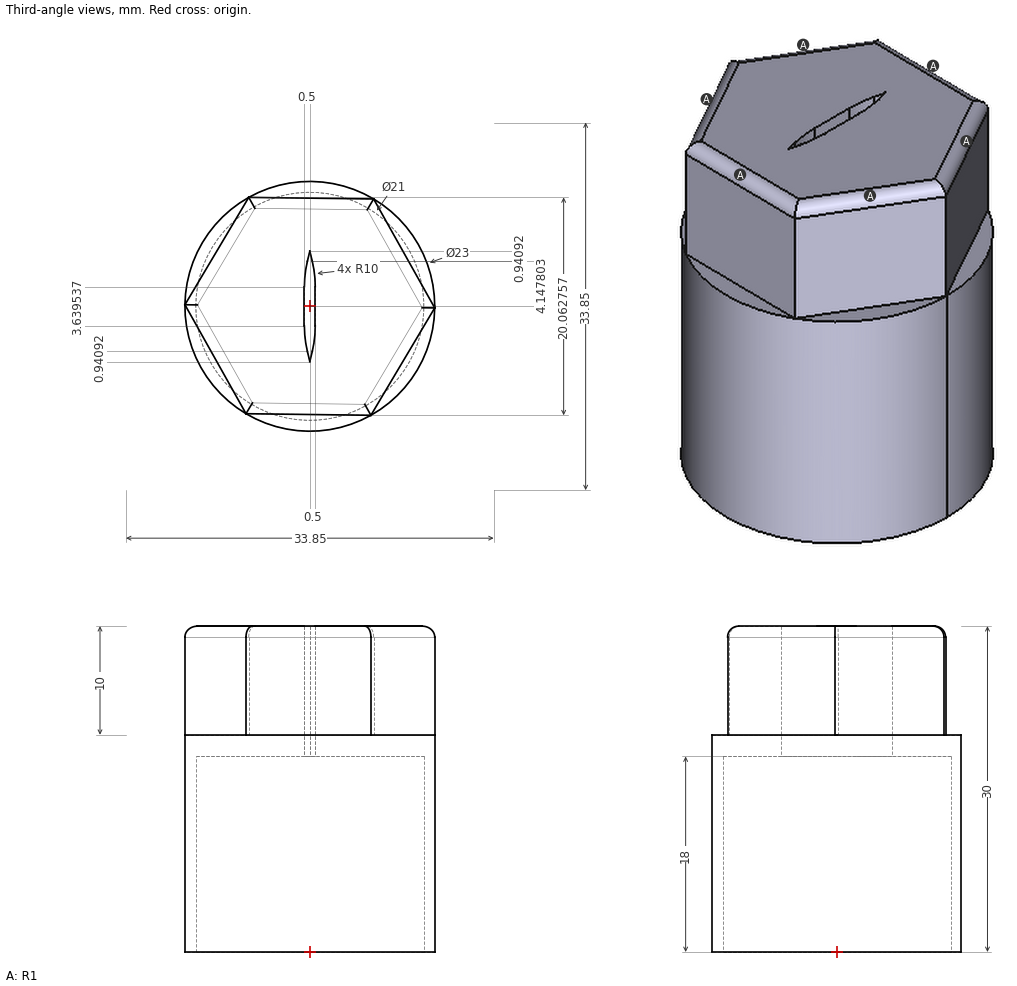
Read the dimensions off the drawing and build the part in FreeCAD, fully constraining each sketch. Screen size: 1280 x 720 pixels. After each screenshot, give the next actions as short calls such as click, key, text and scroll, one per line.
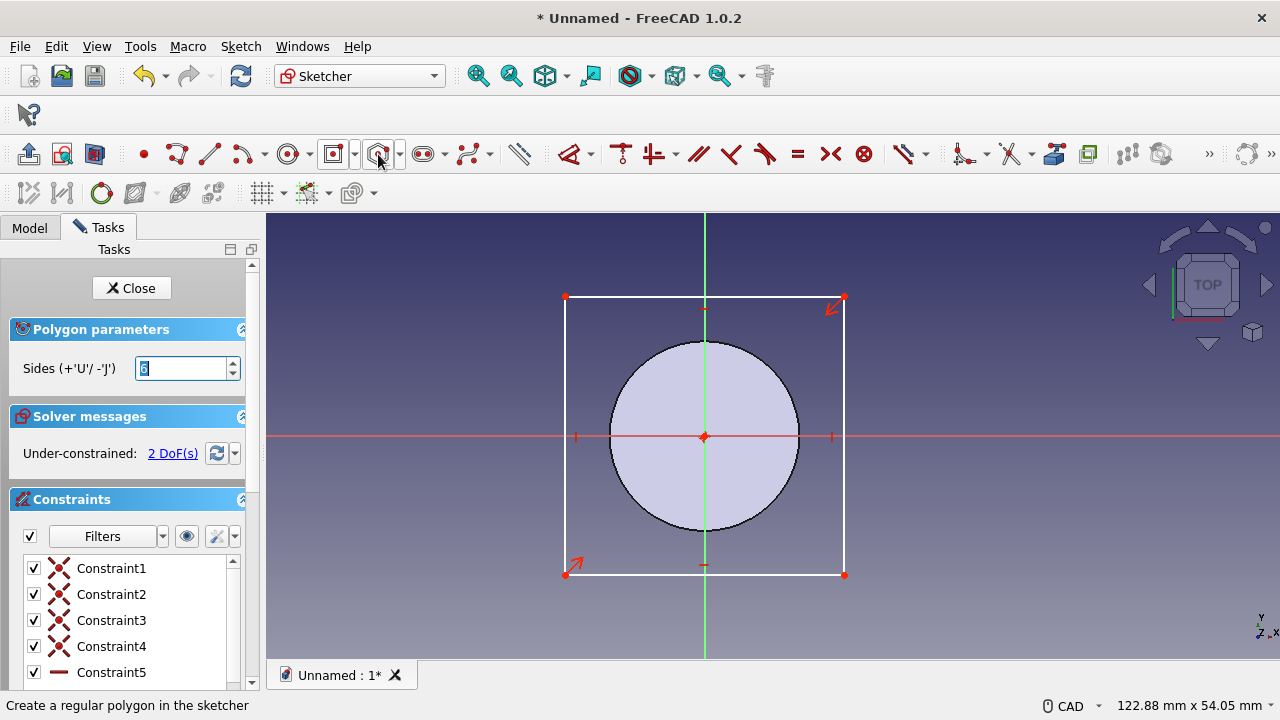
click(705, 436)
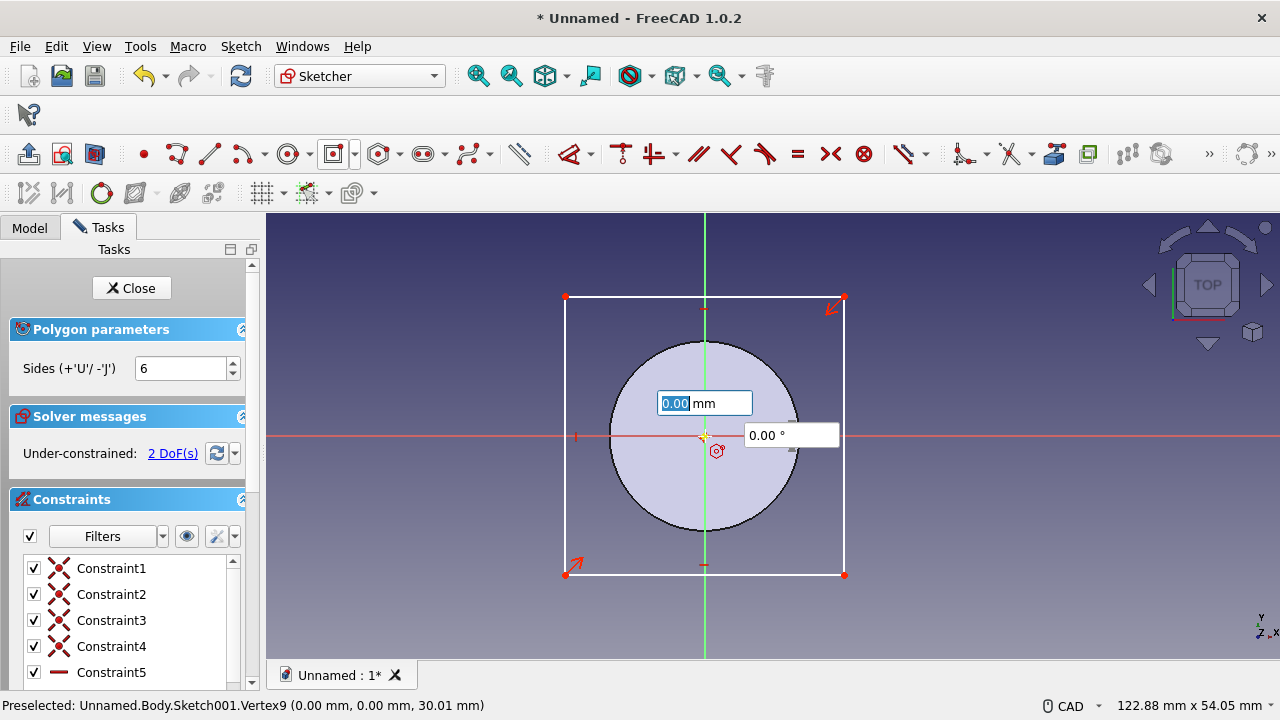
click(753, 355)
key(Escape)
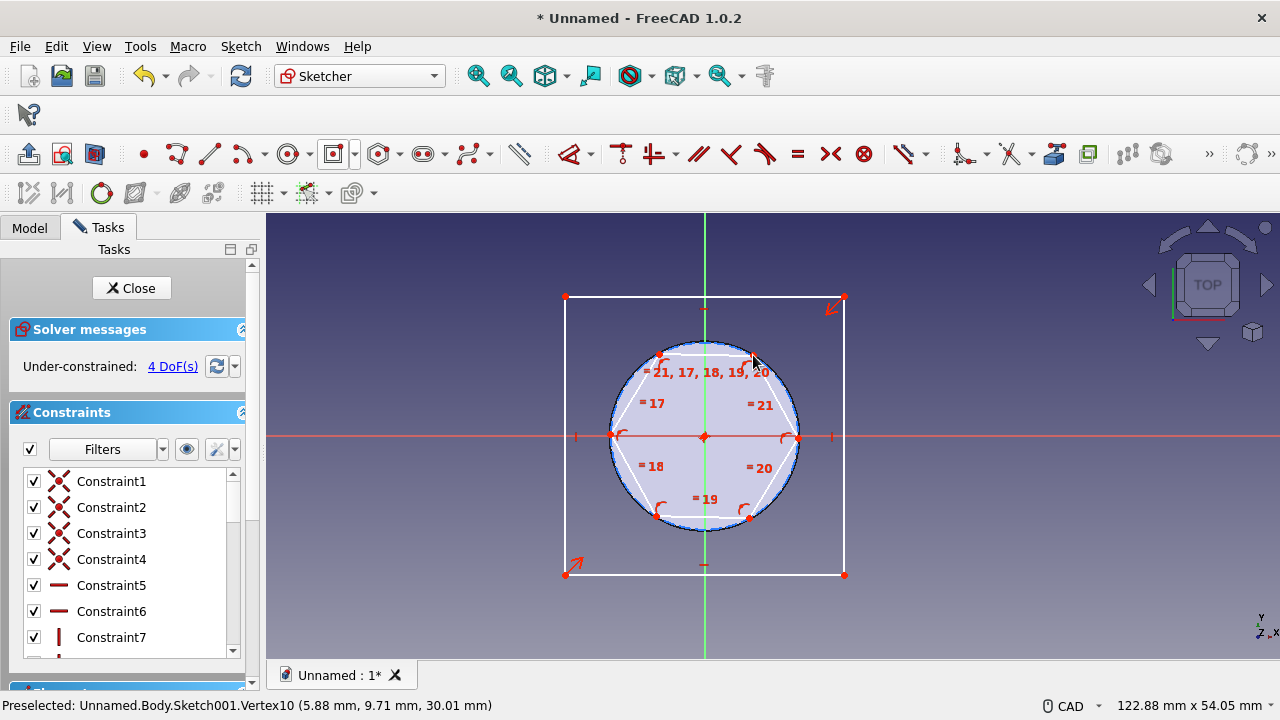
scroll(638, 370, up, 2)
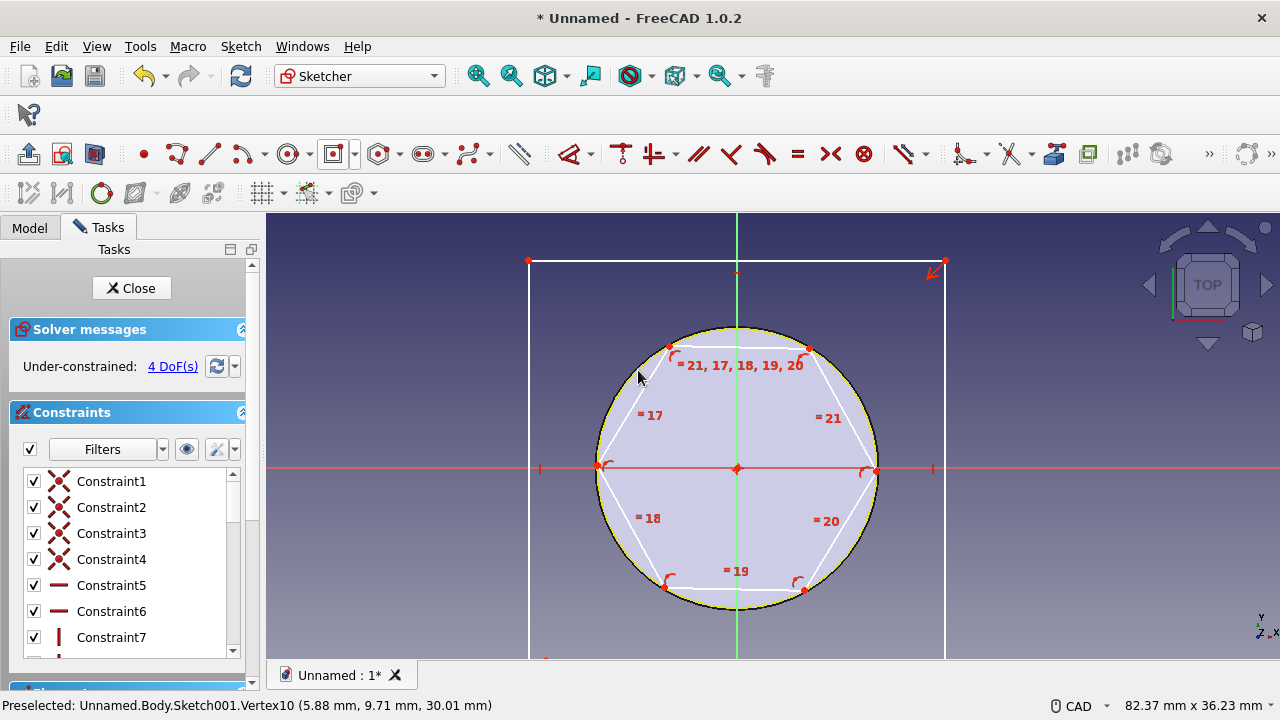
click(638, 370)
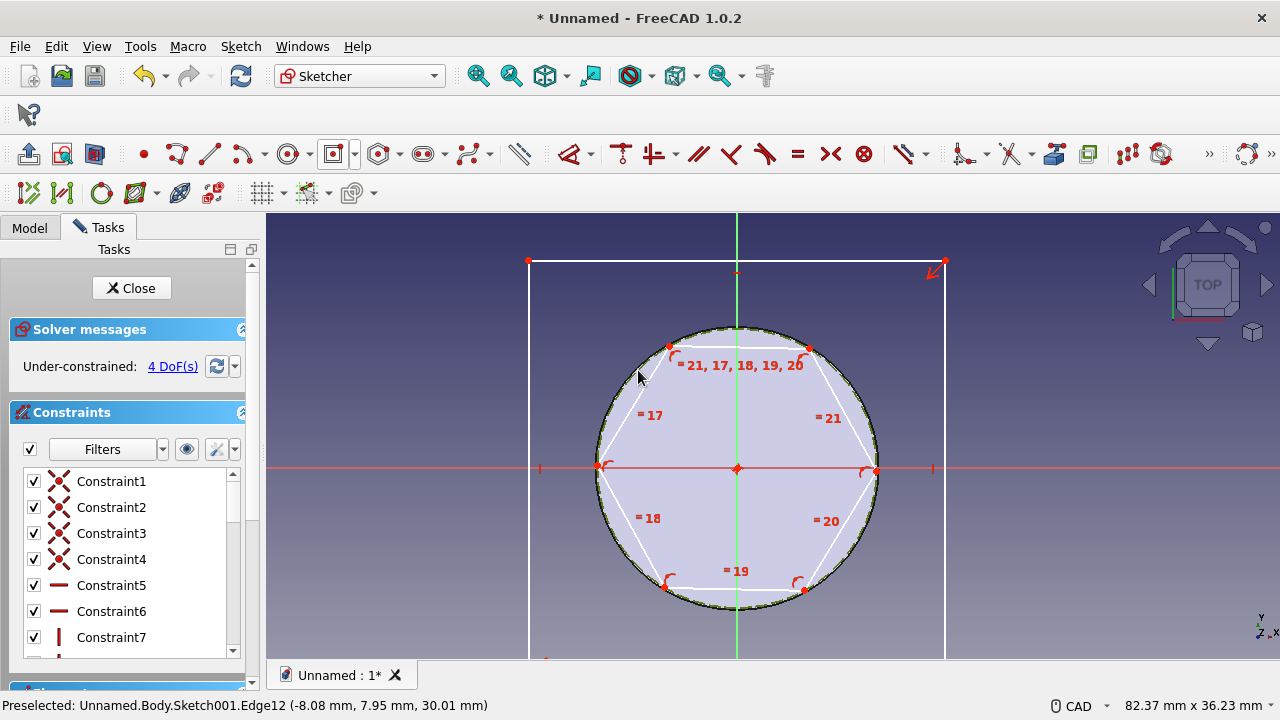
click(590, 154)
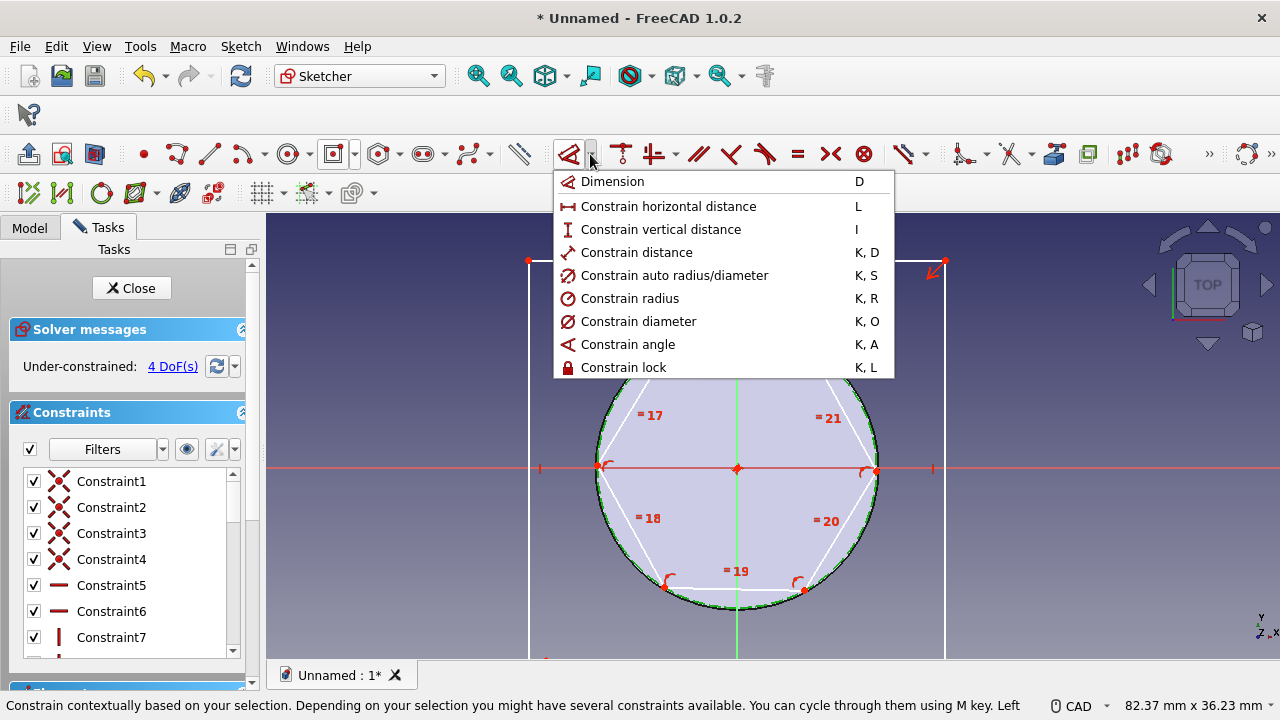
click(724, 322)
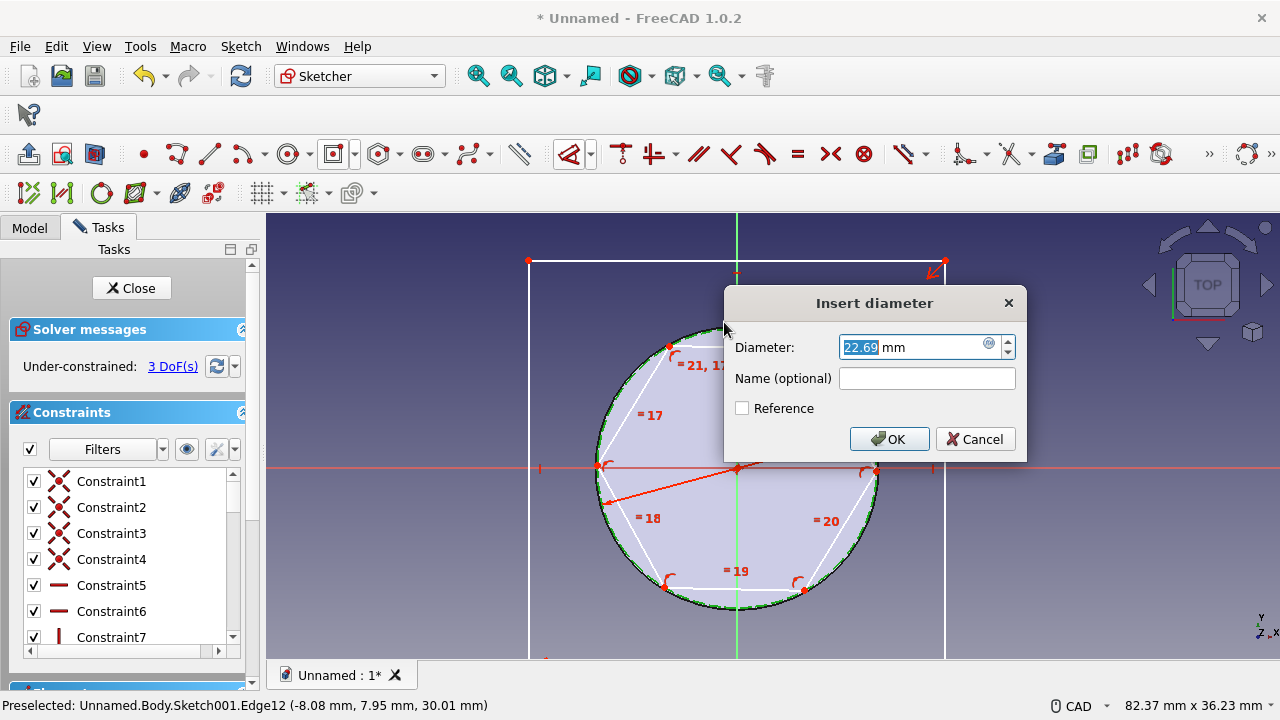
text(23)
key(Return)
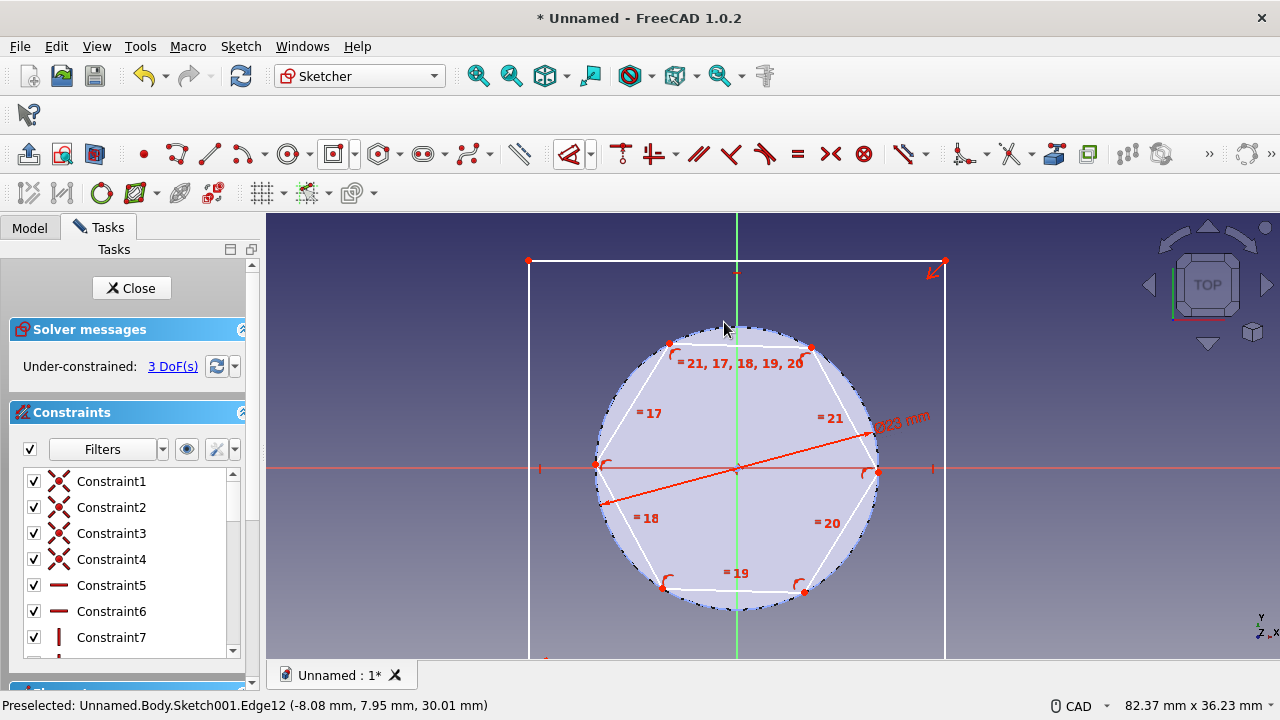
scroll(638, 370, down, 2)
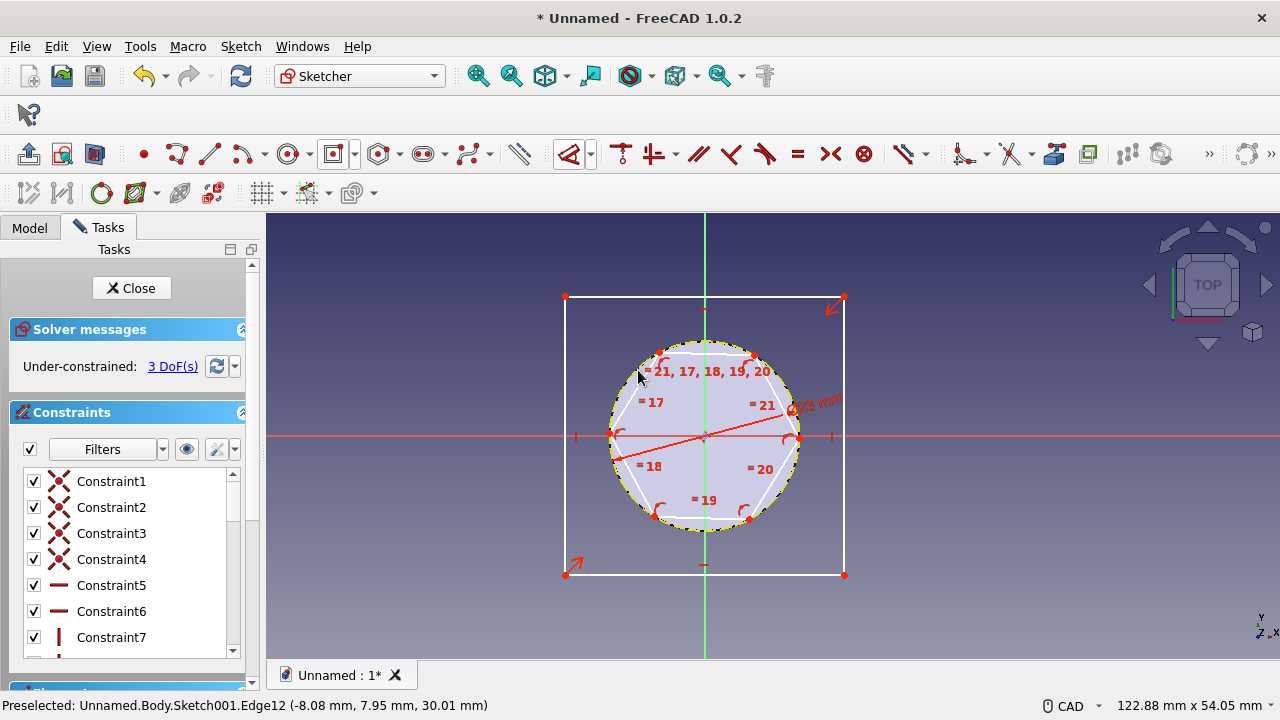
click(649, 575)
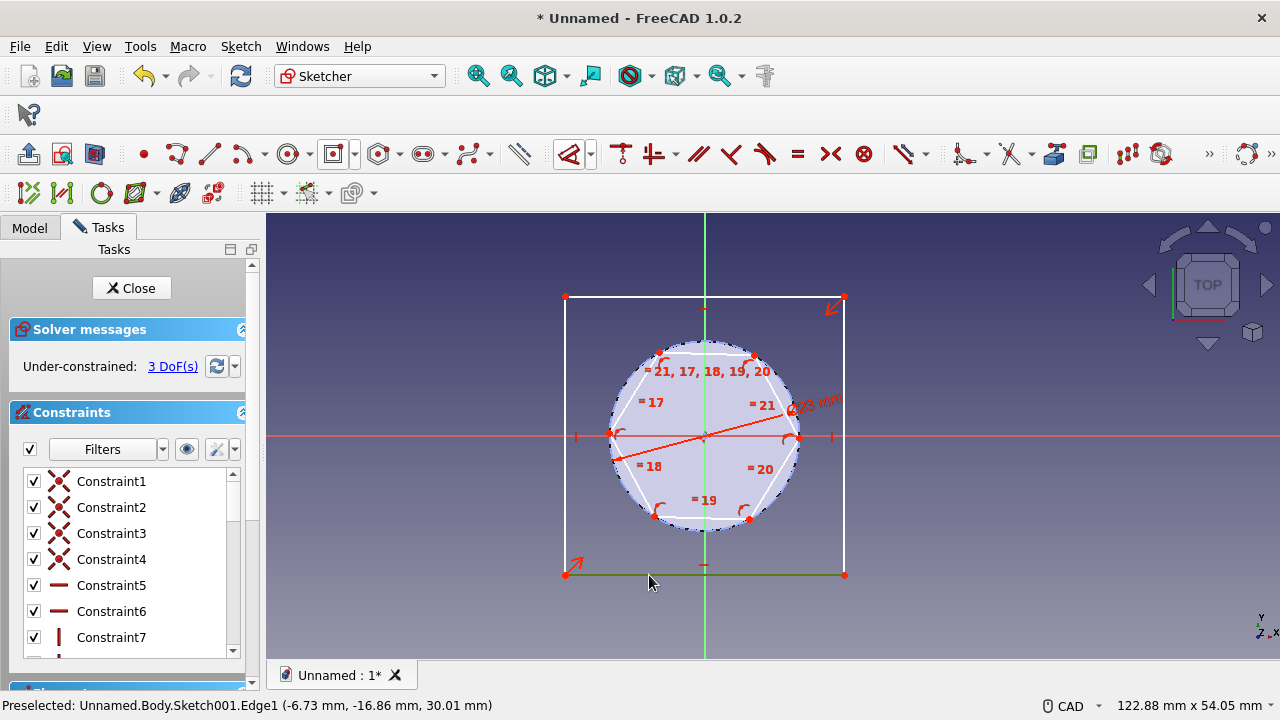
key(l)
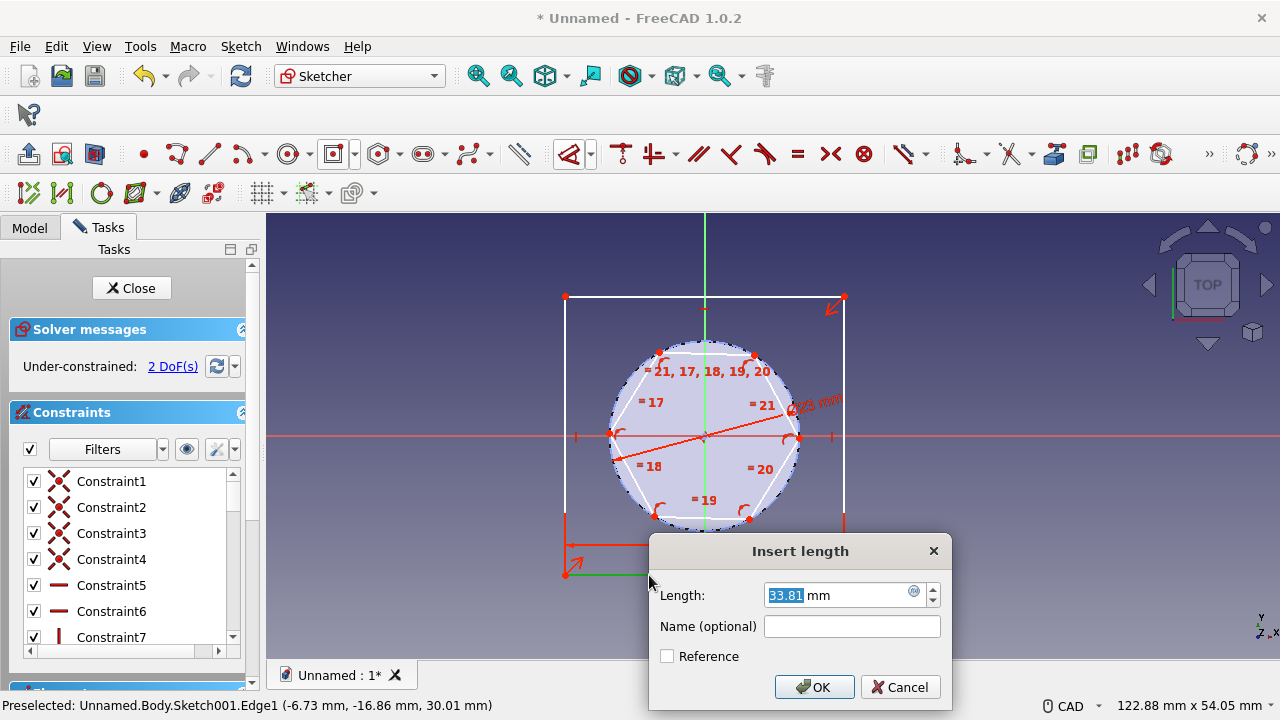
text(33.85)
key(Return)